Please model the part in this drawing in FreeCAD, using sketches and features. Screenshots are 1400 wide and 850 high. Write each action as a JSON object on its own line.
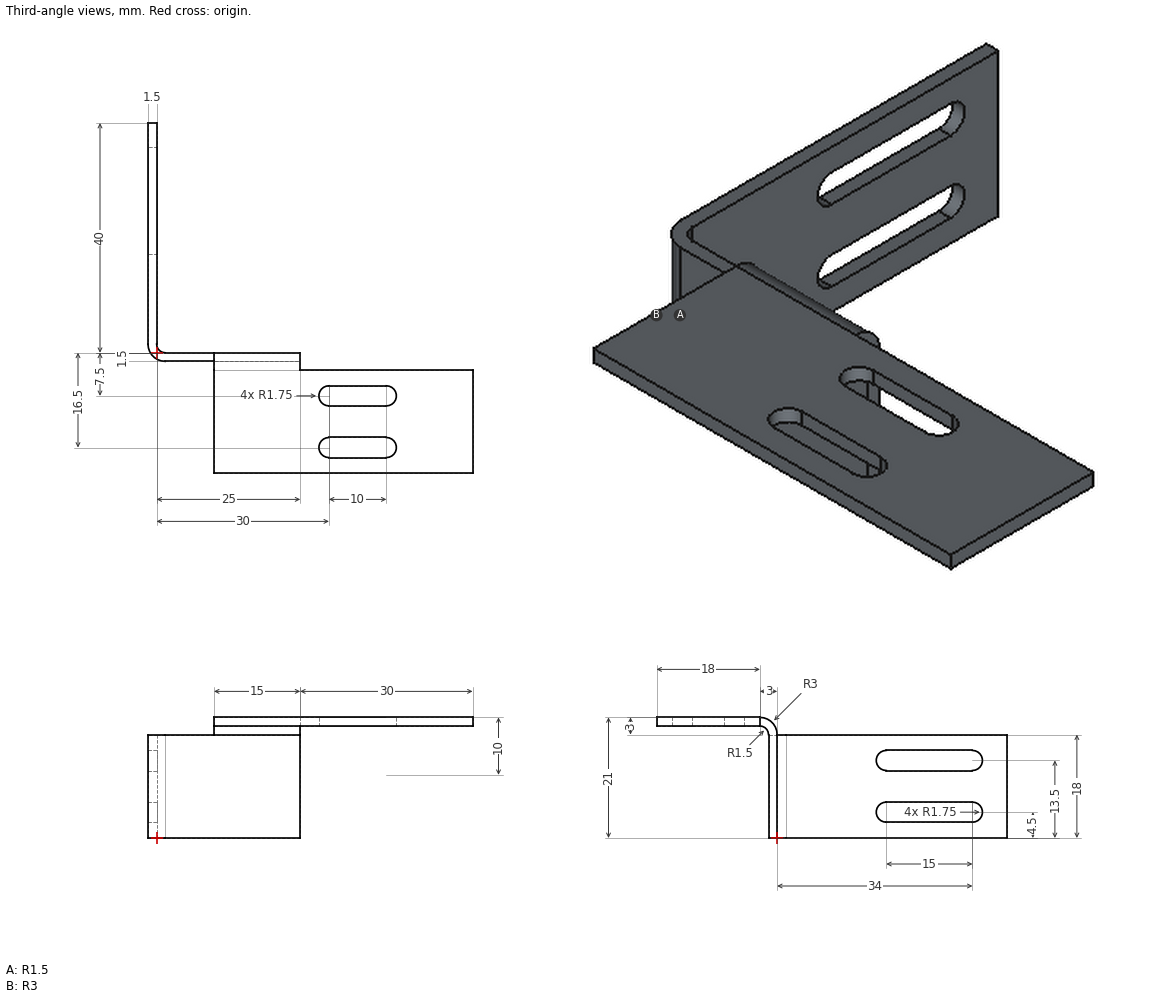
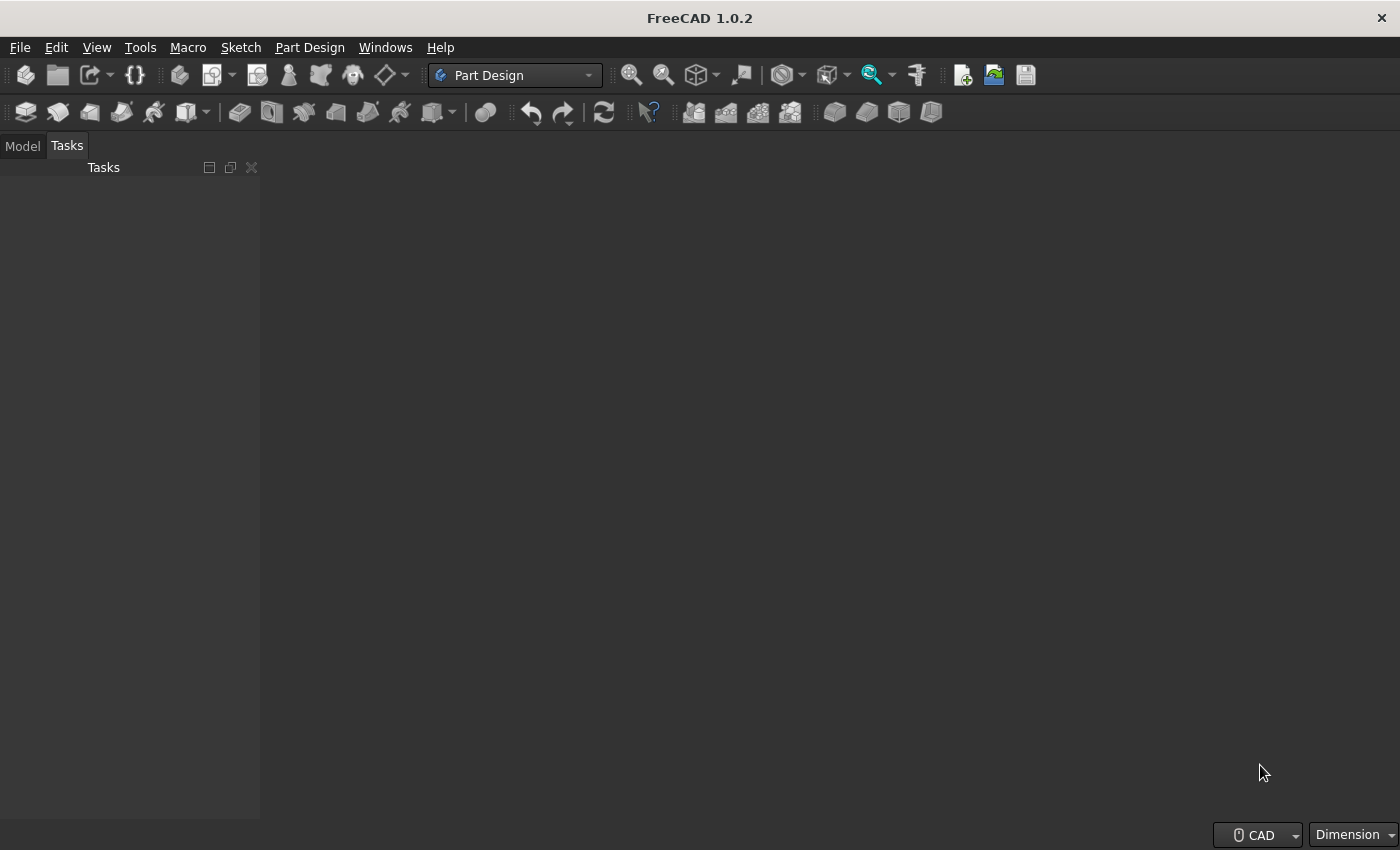
{"action": "left_click", "coordinate": [962, 76]}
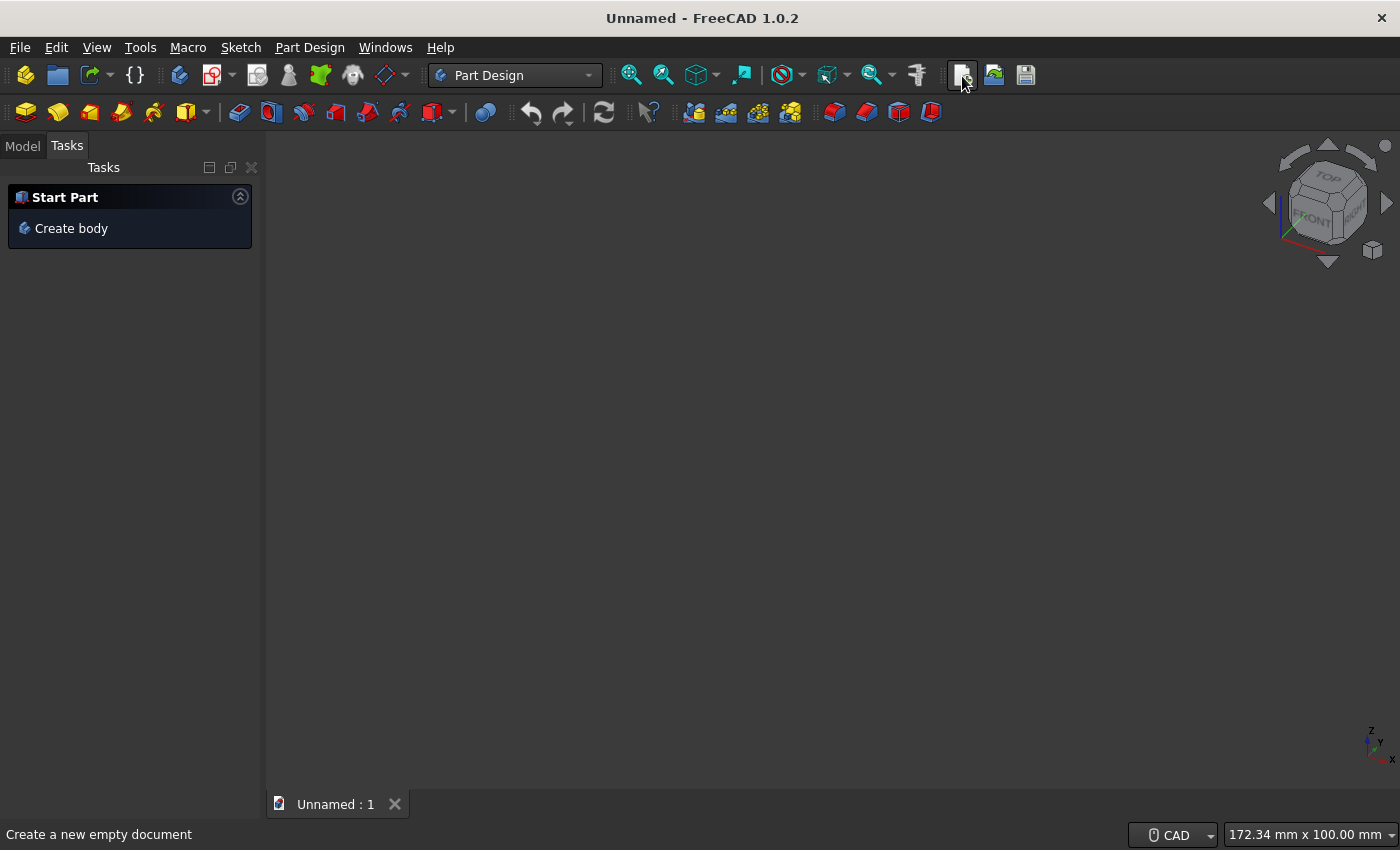
{"action": "left_click", "coordinate": [212, 76]}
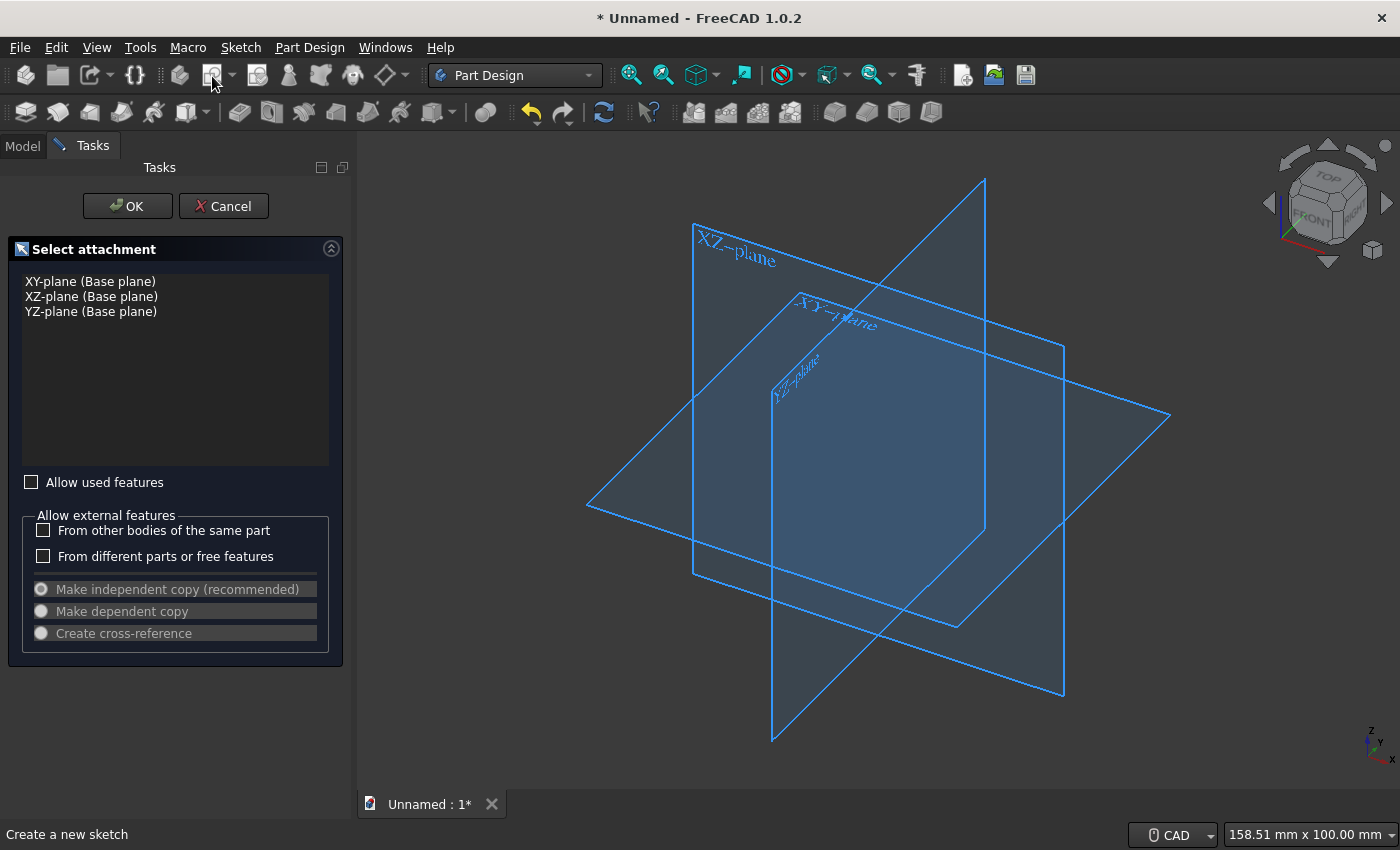
{"action": "left_click", "coordinate": [82, 282]}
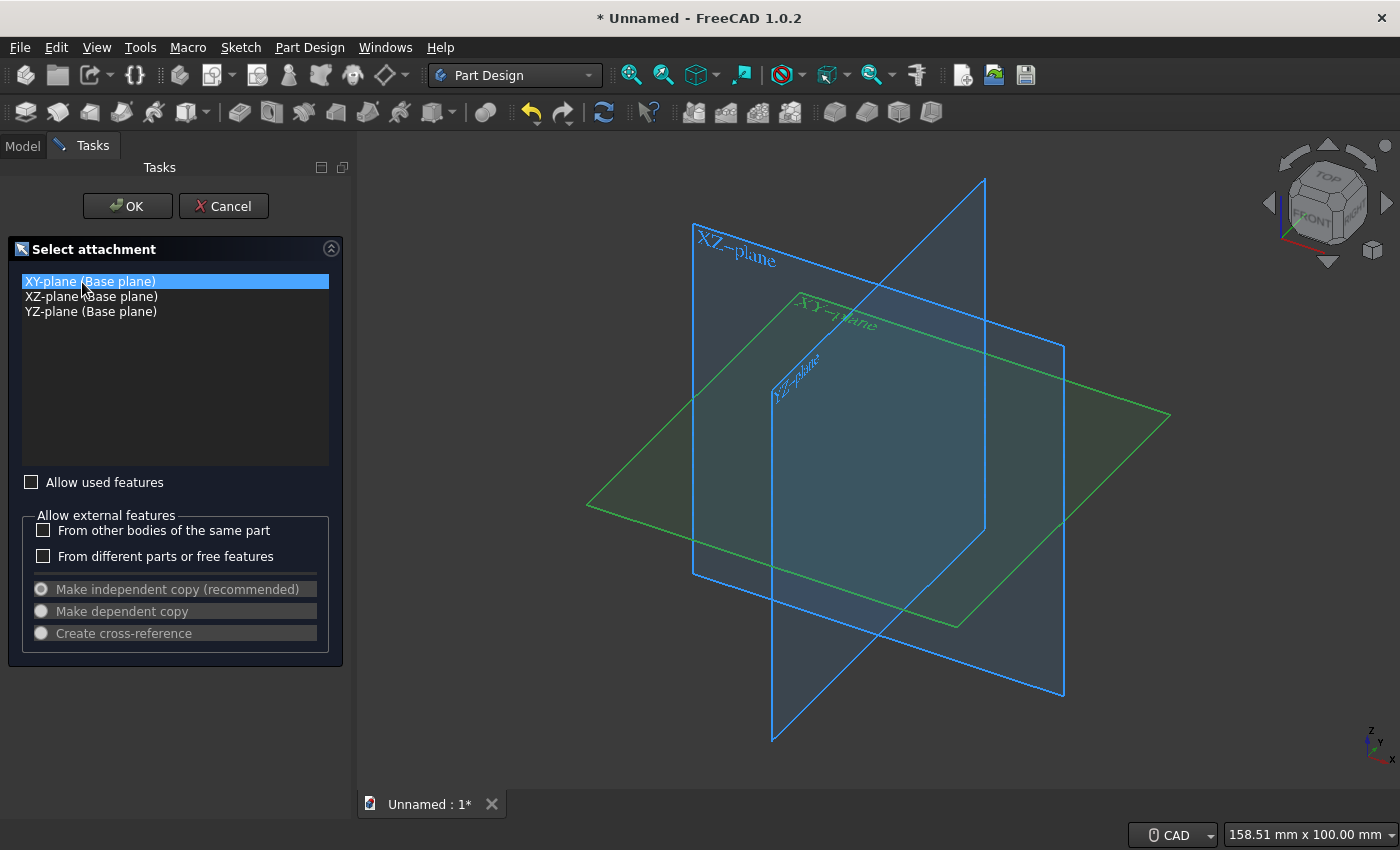
{"action": "left_click", "coordinate": [128, 206]}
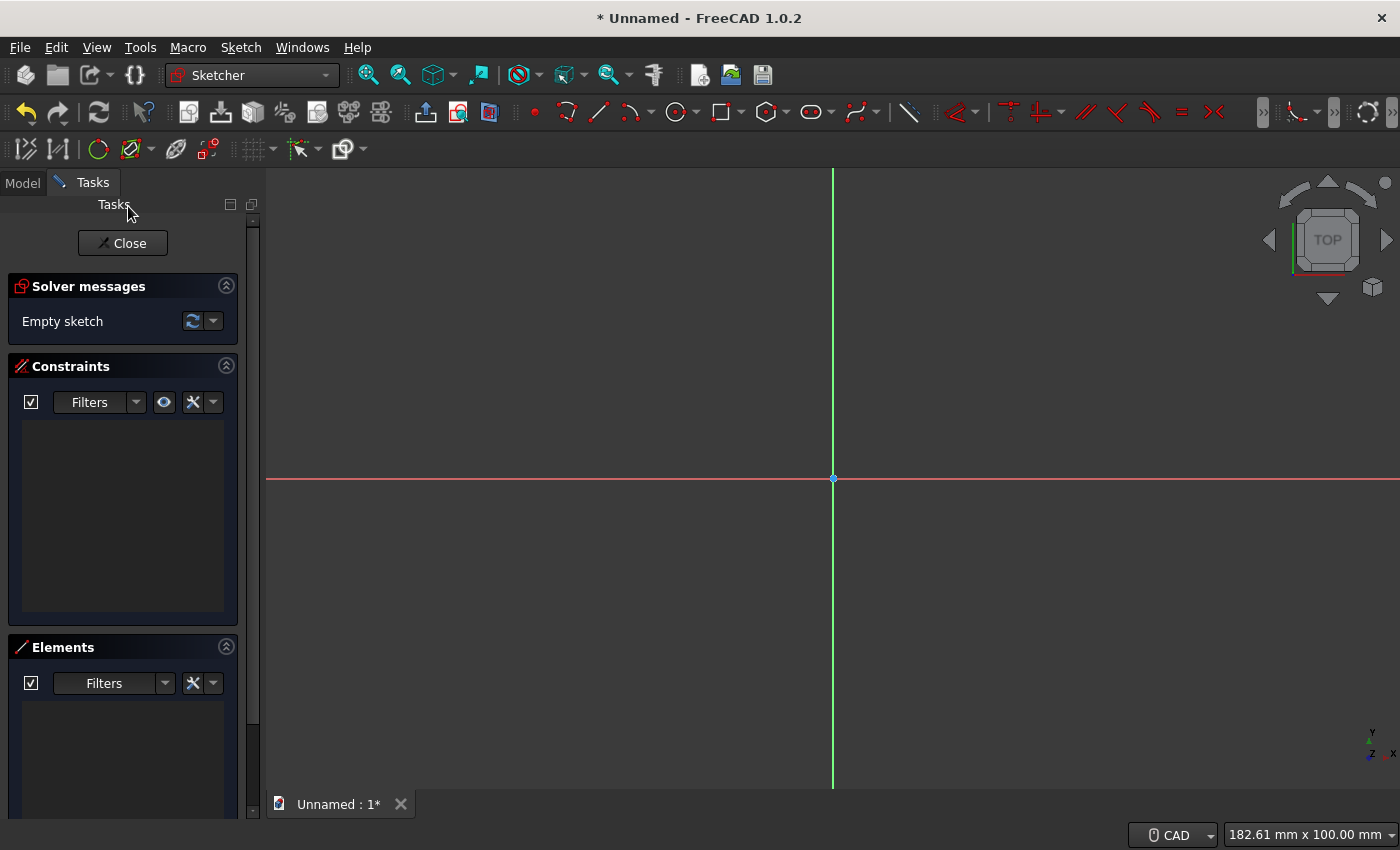
{"action": "scroll", "coordinate": [1194, 196], "scroll_direction": "up", "scroll_amount": 2}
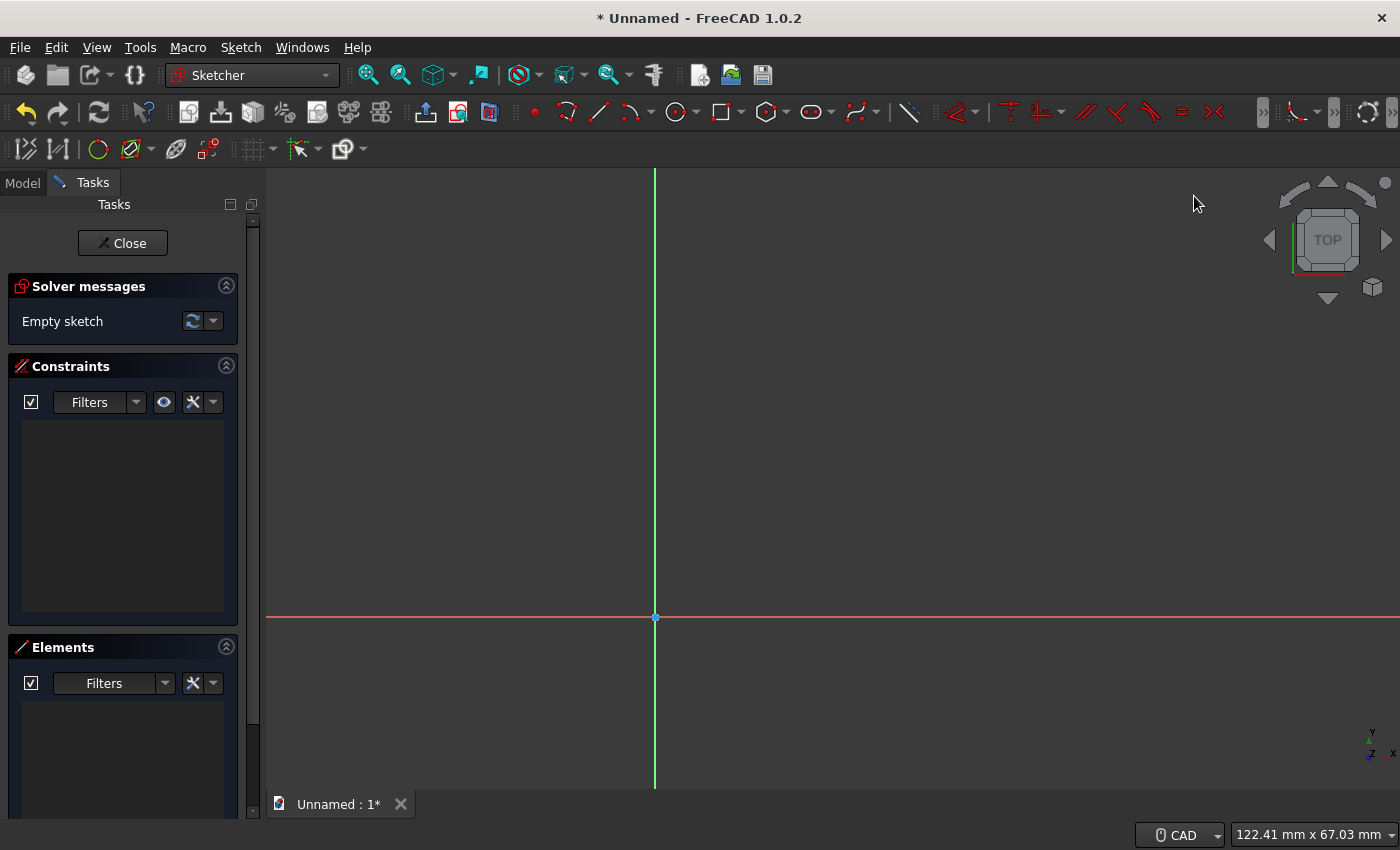
{"action": "key", "text": "g m"}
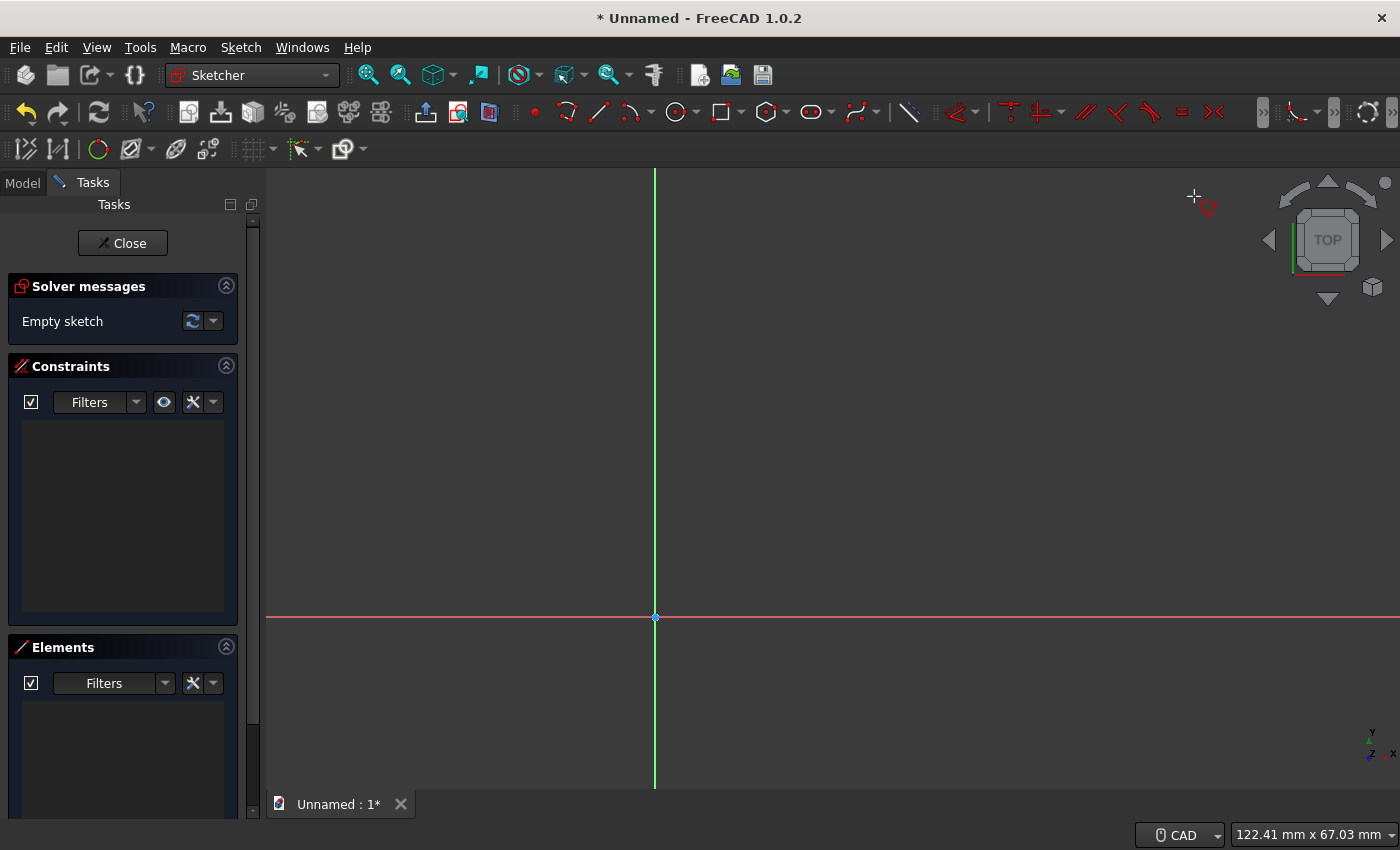
{"action": "left_click", "coordinate": [655, 617]}
{"action": "left_click", "coordinate": [664, 247]}
{"action": "left_click", "coordinate": [641, 247]}
{"action": "left_click", "coordinate": [641, 631]}
{"action": "left_click", "coordinate": [887, 631]}
{"action": "left_click", "coordinate": [887, 608]}
{"action": "left_click", "coordinate": [655, 617]}
{"action": "key", "text": "Escape"}
{"action": "key", "text": "Escape"}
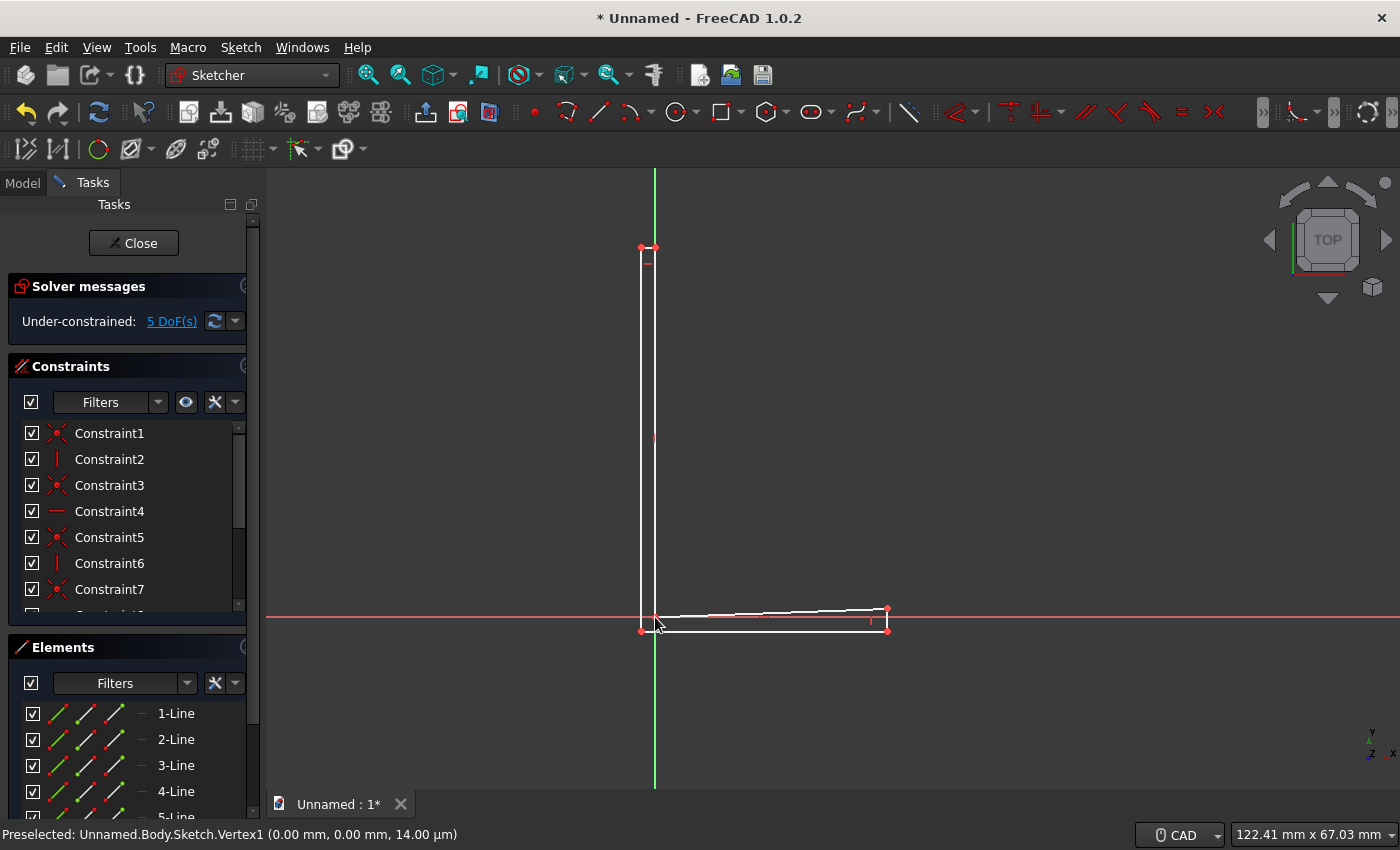
{"action": "left_click", "coordinate": [725, 615]}